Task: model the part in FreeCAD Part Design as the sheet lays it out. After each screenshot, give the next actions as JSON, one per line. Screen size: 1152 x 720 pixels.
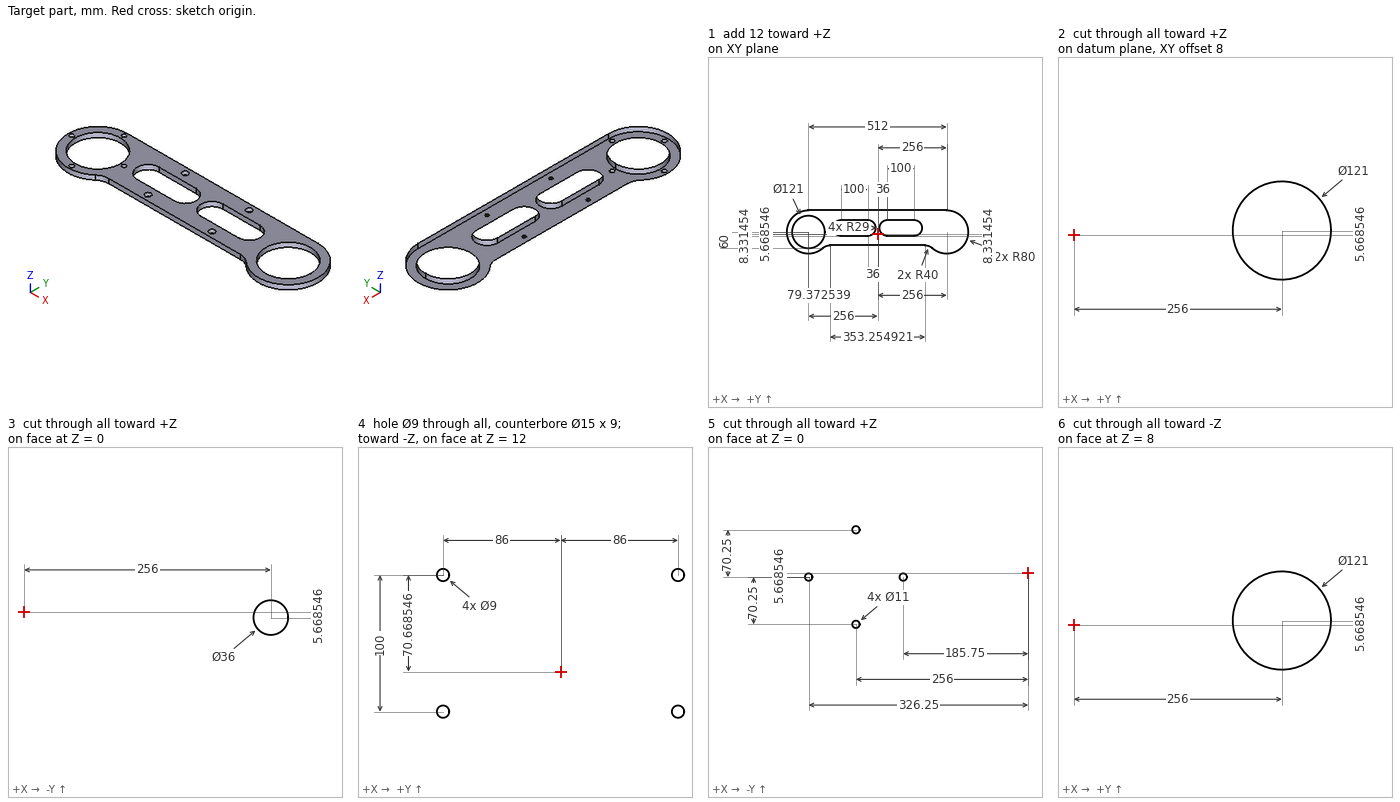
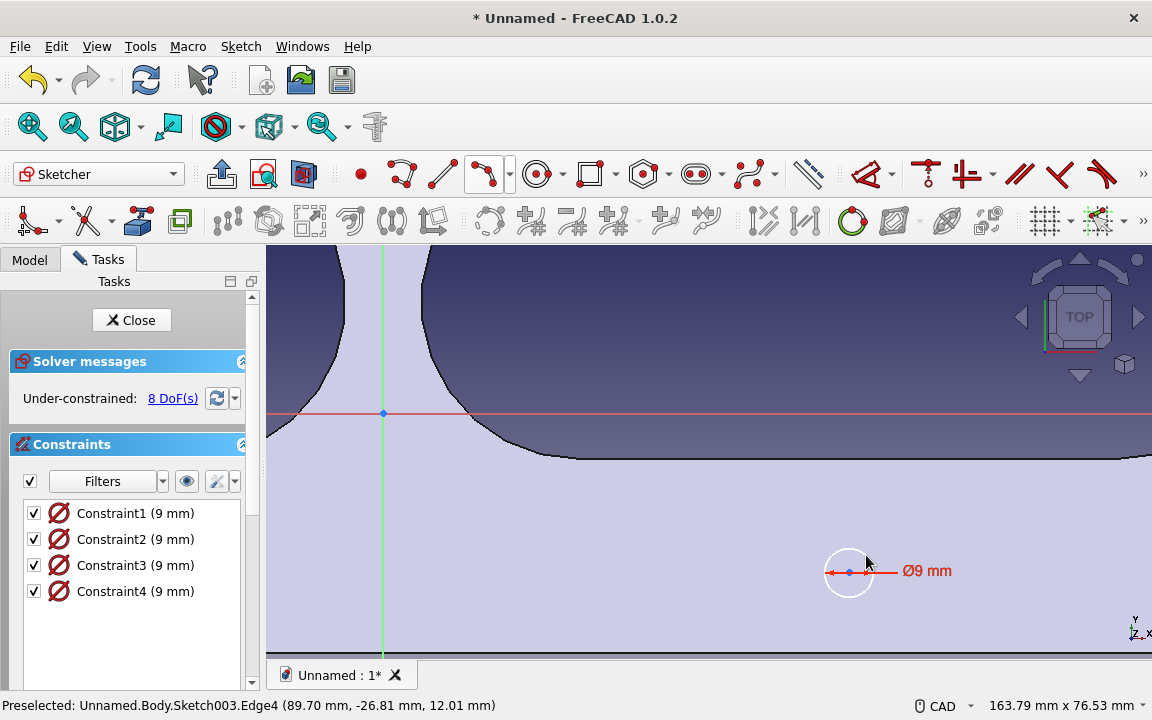
{"action": "scroll", "coordinate": [850, 574], "scroll_direction": "down", "scroll_amount": 4}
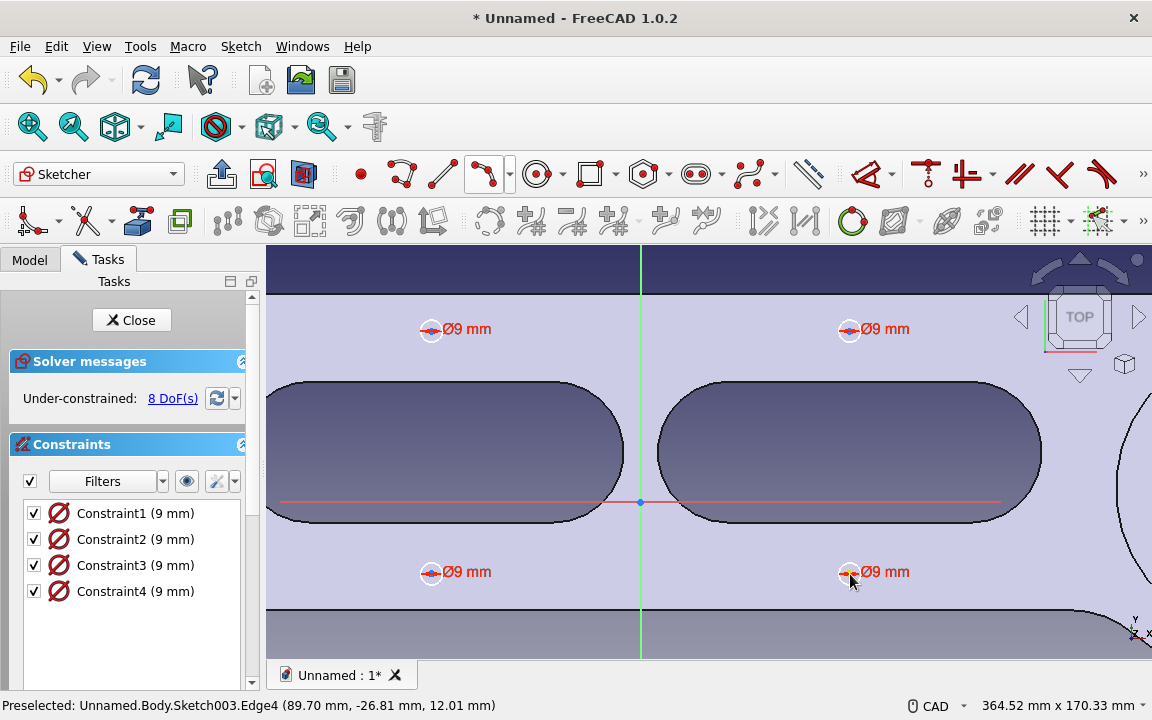
{"action": "left_click", "coordinate": [432, 331]}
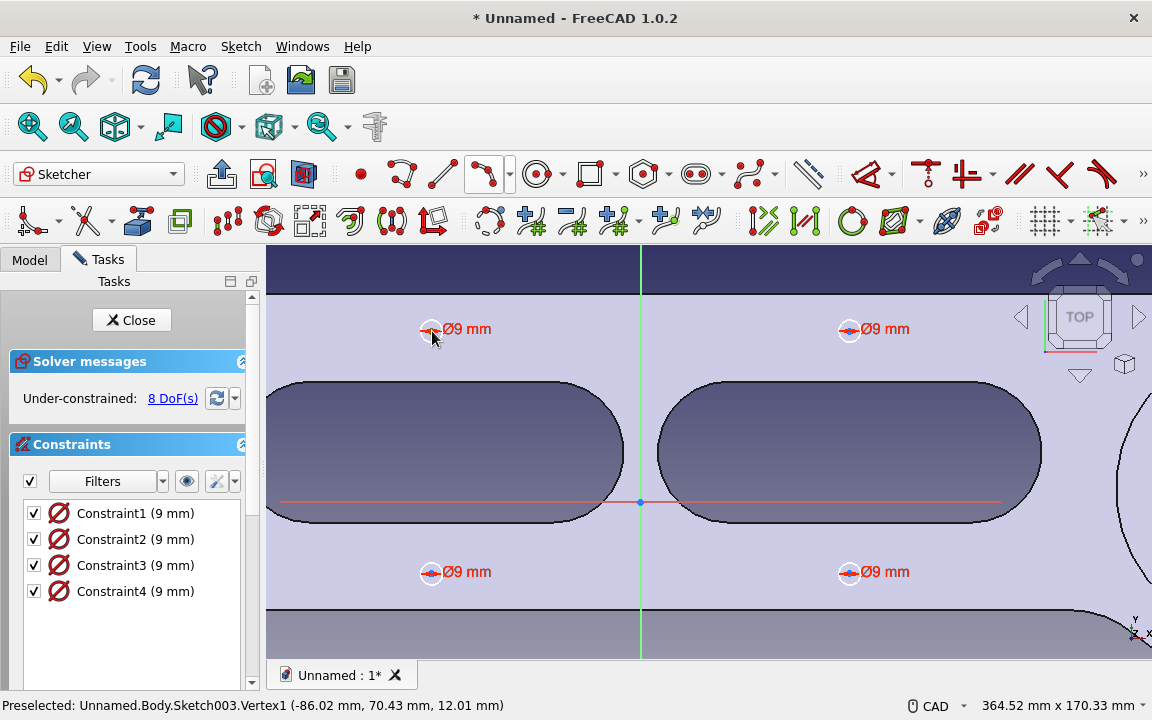
{"action": "left_click", "coordinate": [432, 574]}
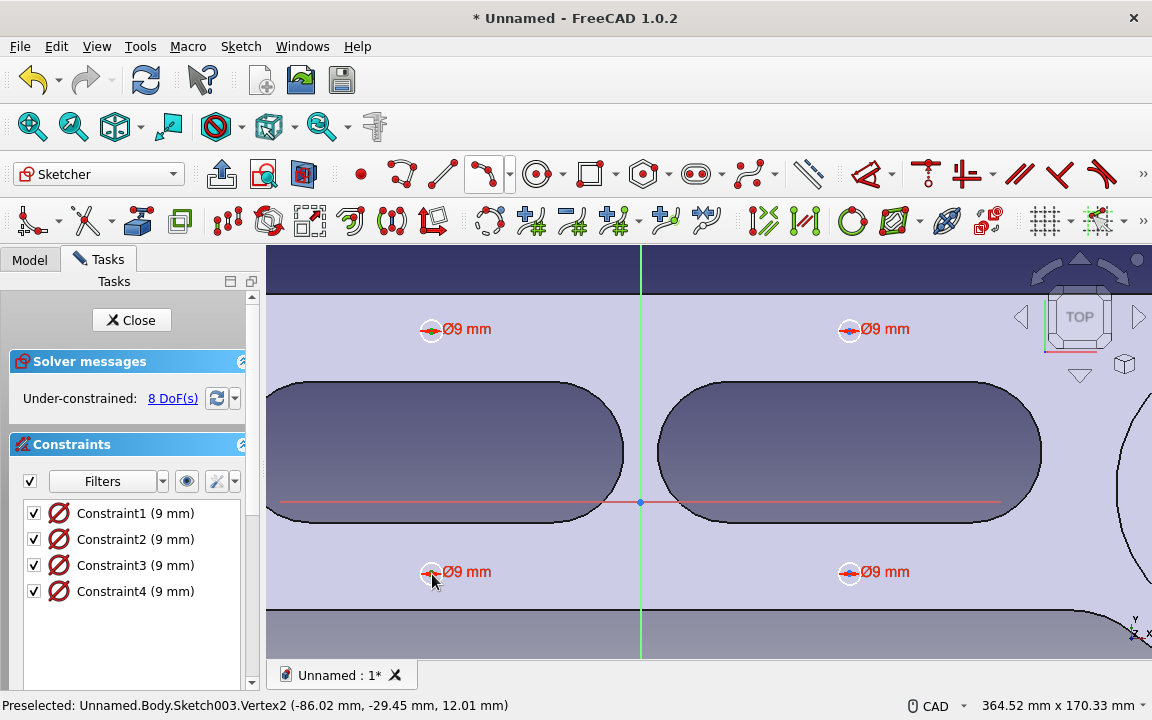
{"action": "left_click", "coordinate": [992, 174]}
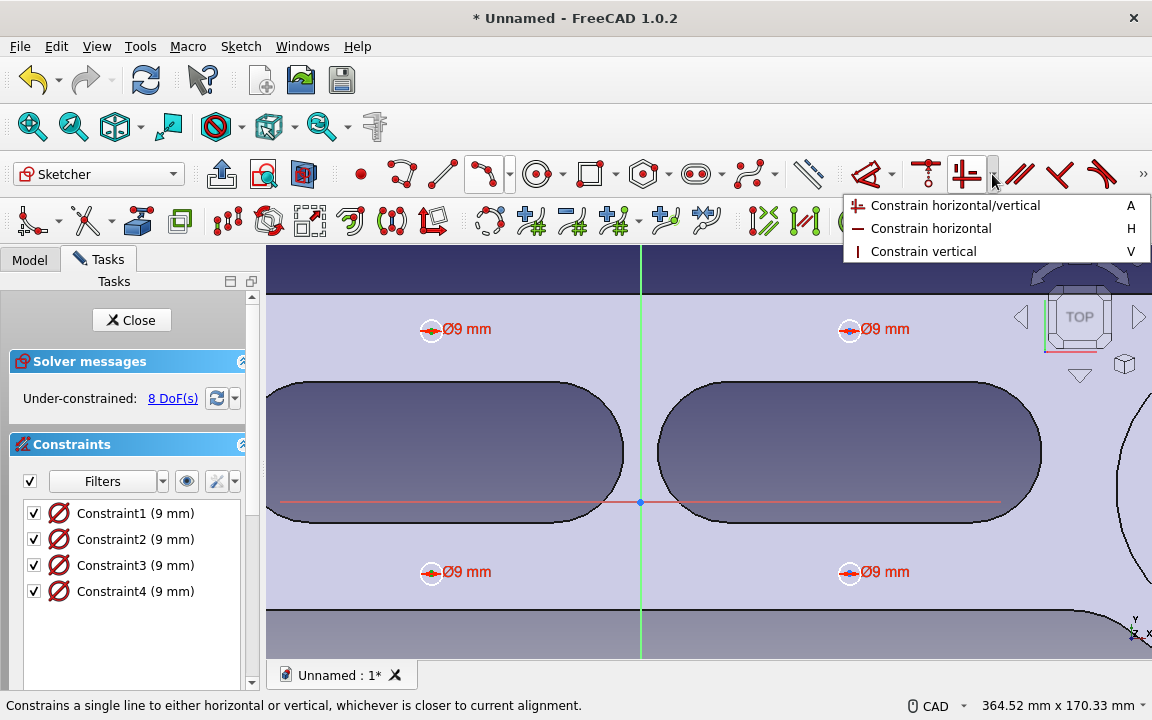
{"action": "left_click", "coordinate": [997, 252]}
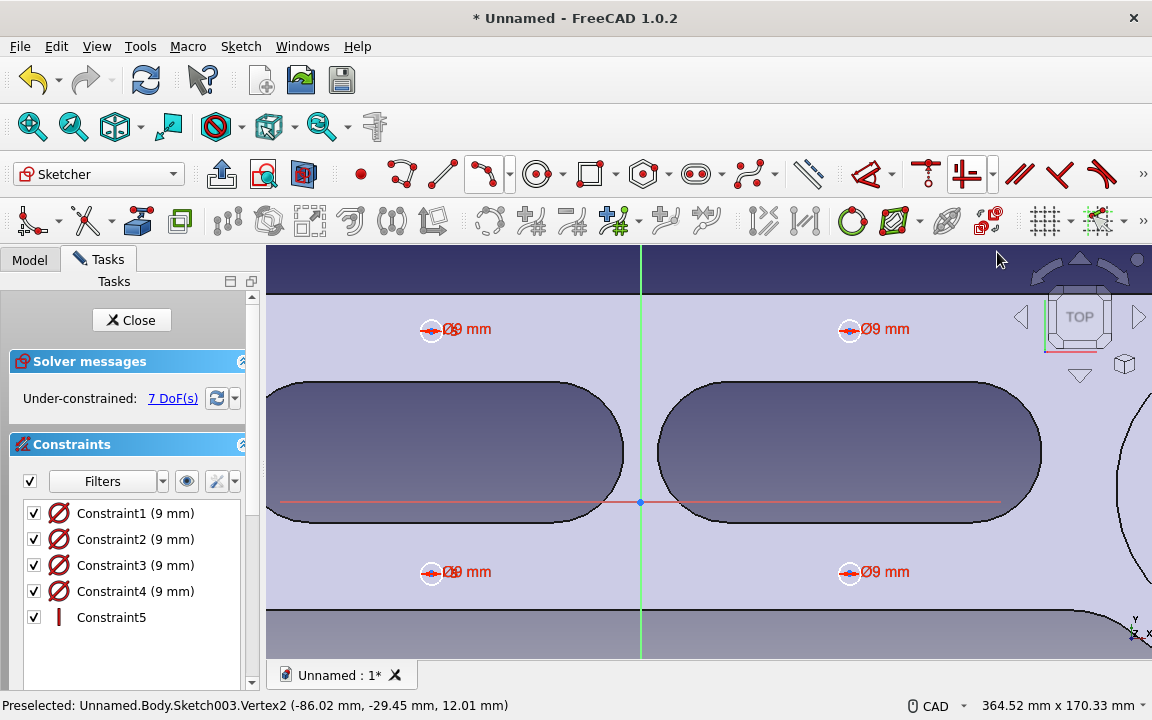
{"action": "left_click", "coordinate": [432, 331]}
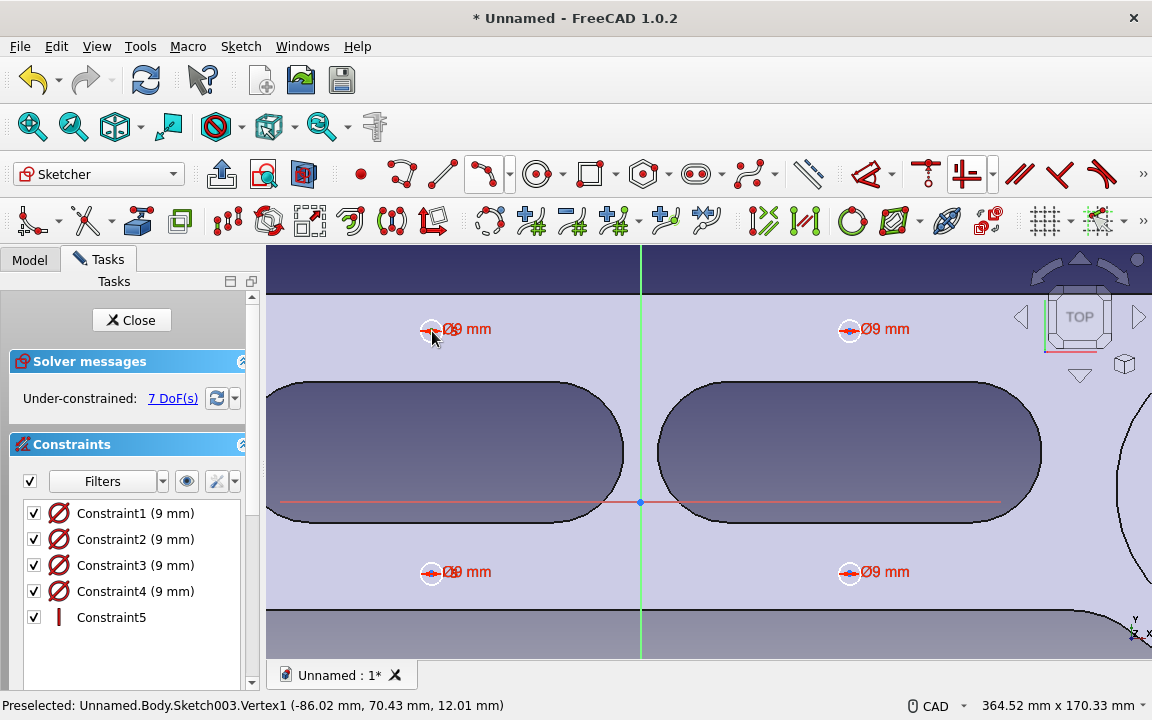
{"action": "left_click", "coordinate": [850, 331]}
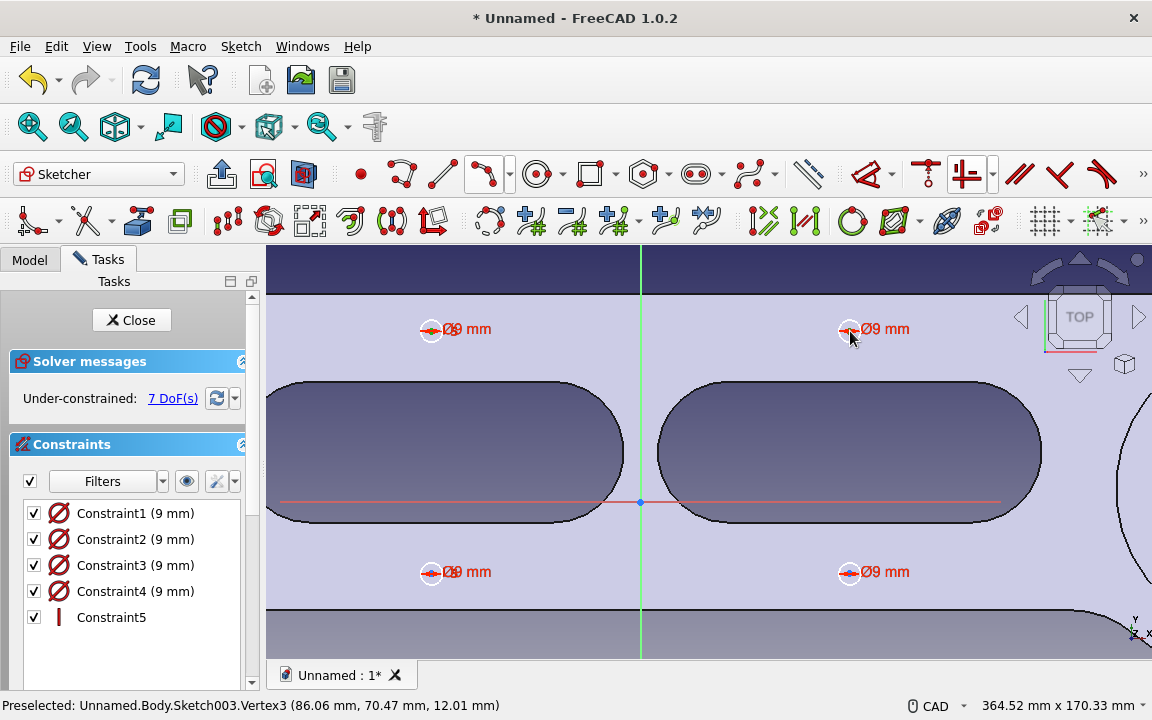
{"action": "key", "text": "h"}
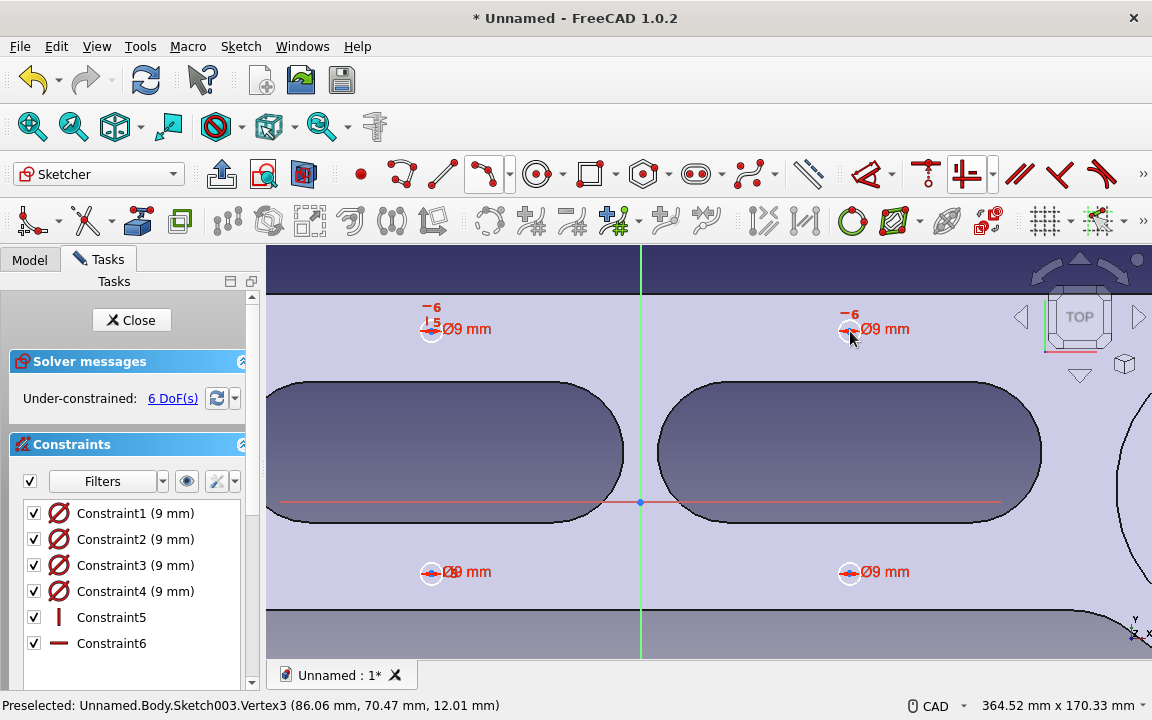
{"action": "left_click", "coordinate": [850, 331]}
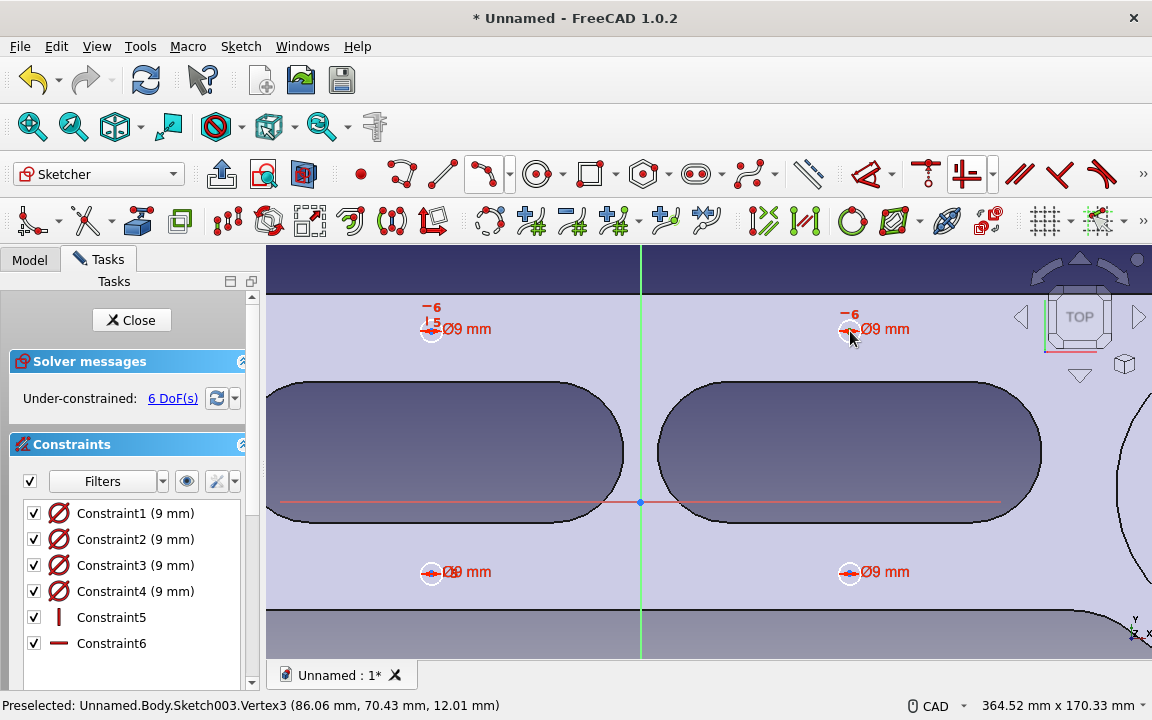
{"action": "left_click", "coordinate": [850, 574]}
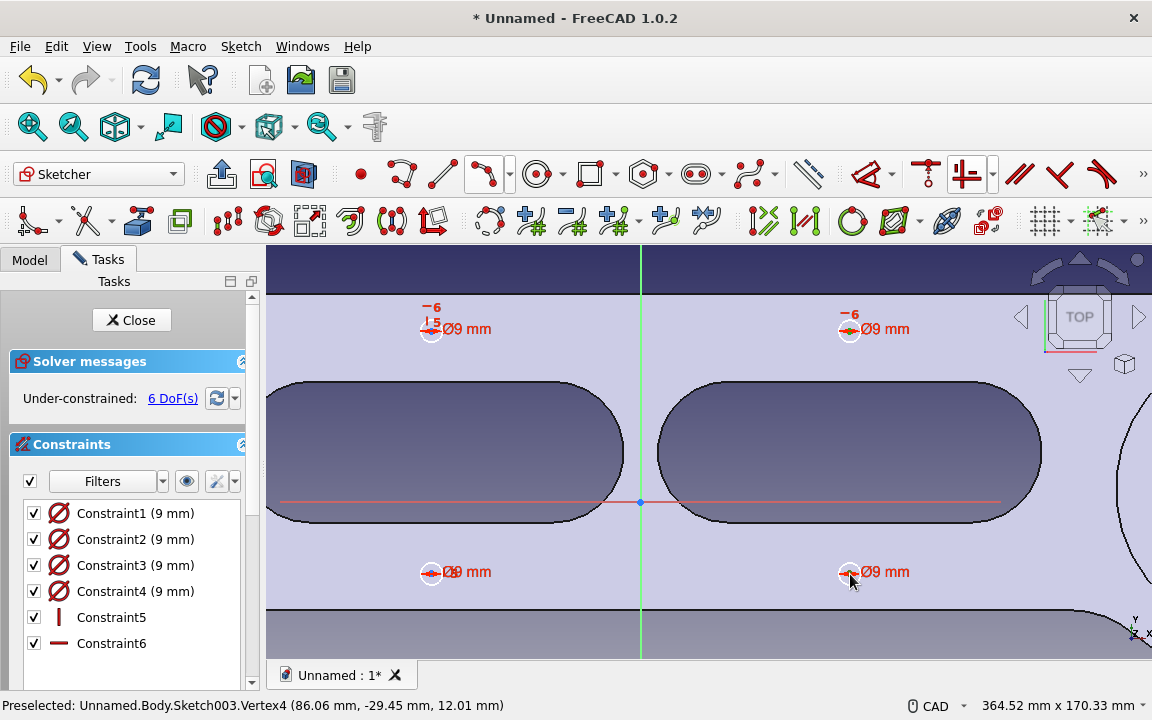
{"action": "left_click", "coordinate": [992, 174]}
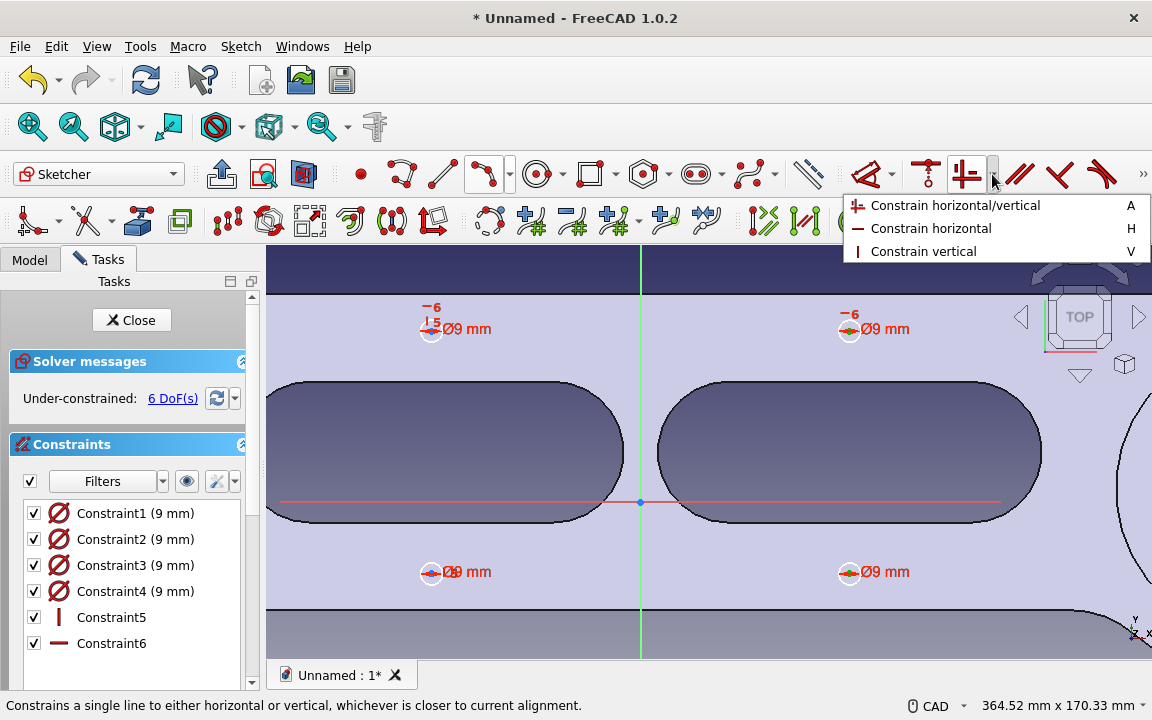
{"action": "left_click", "coordinate": [997, 252]}